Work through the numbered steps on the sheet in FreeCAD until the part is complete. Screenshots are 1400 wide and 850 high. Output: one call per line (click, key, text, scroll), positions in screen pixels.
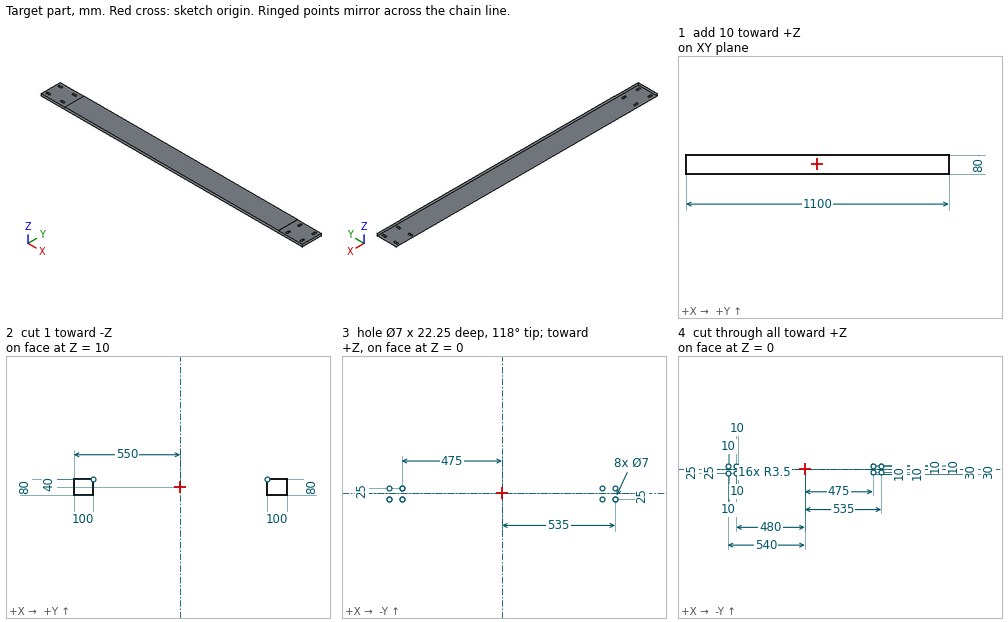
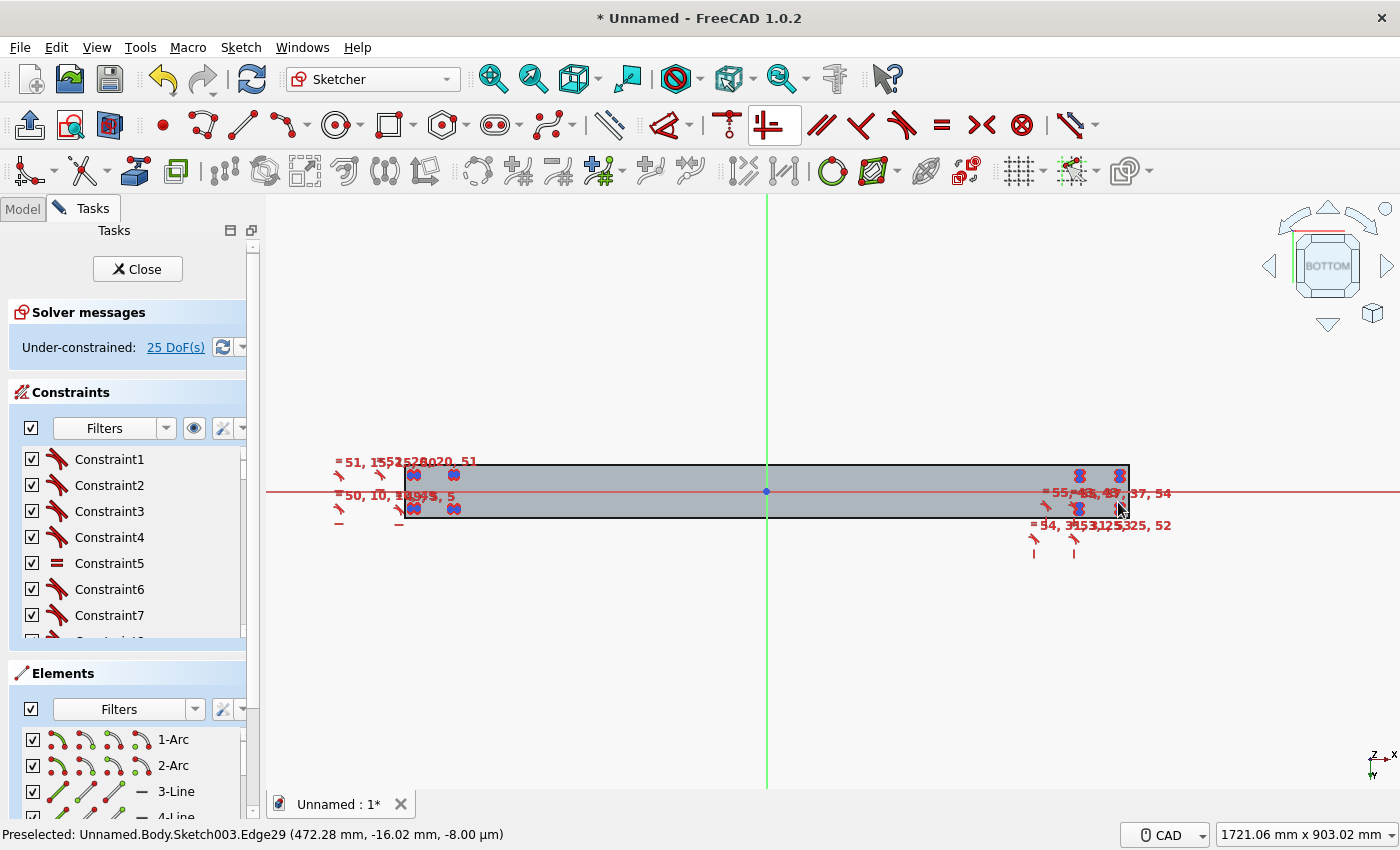
scroll(411, 508, up, 8)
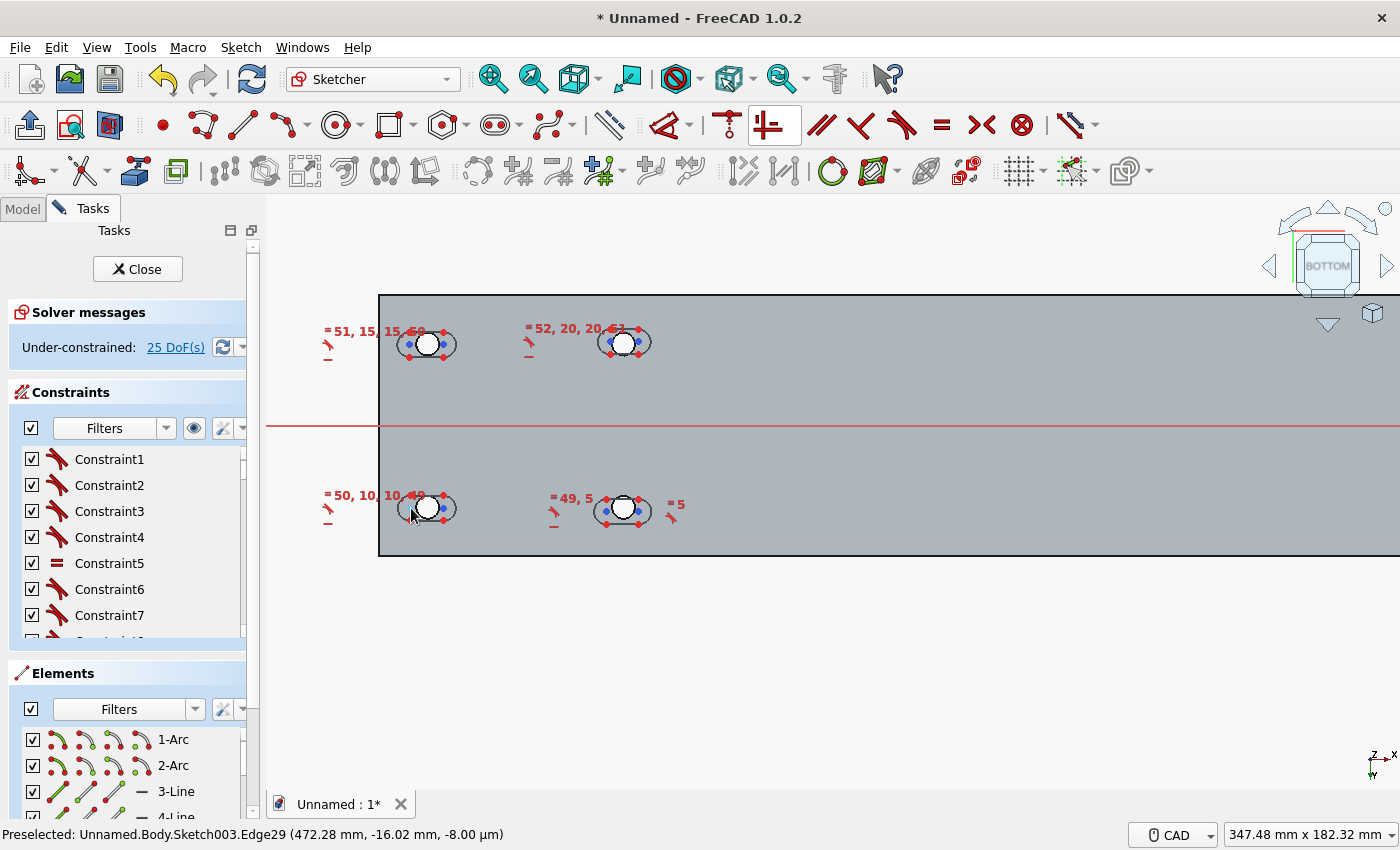
click(410, 508)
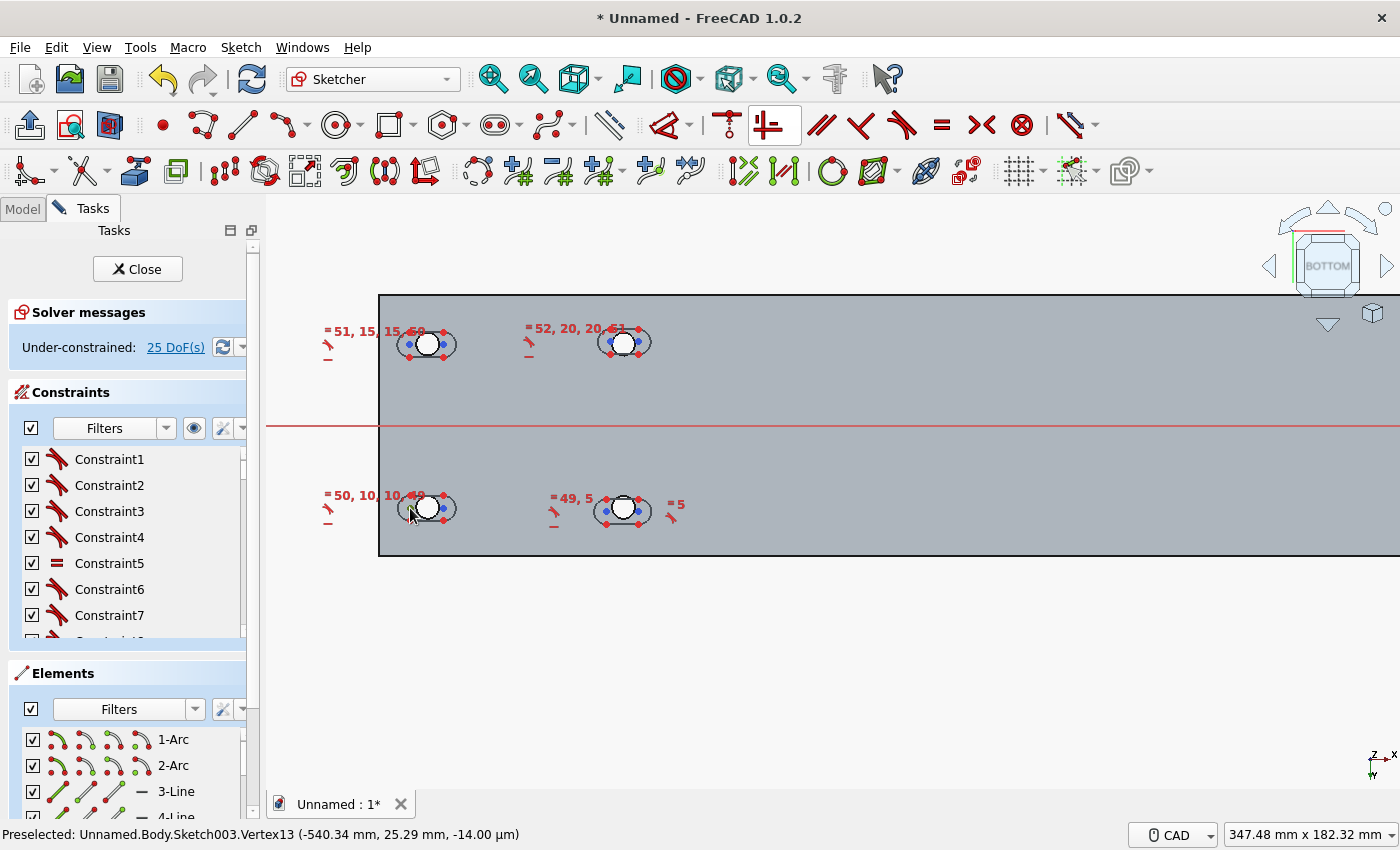
click(410, 345)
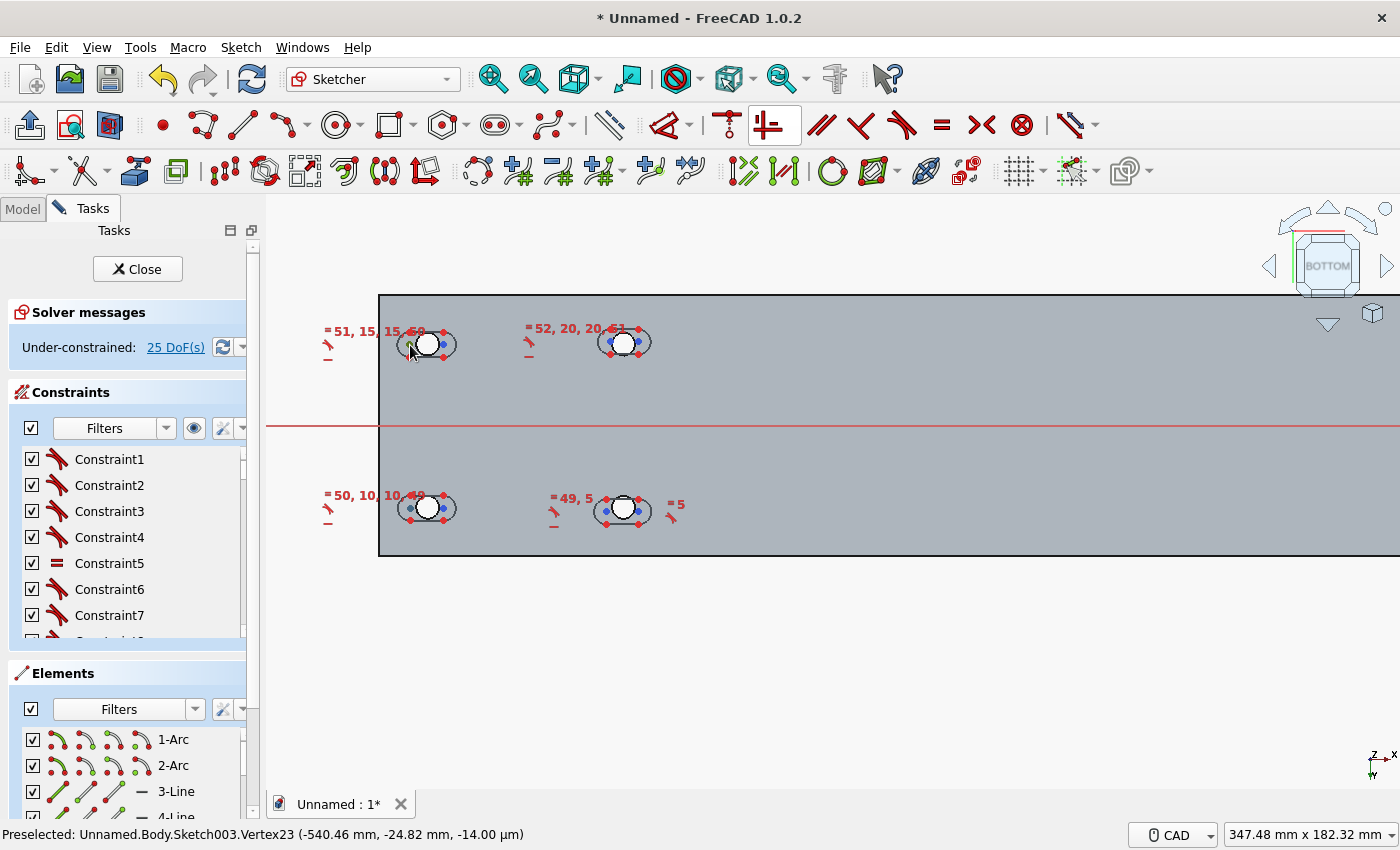
click(361, 426)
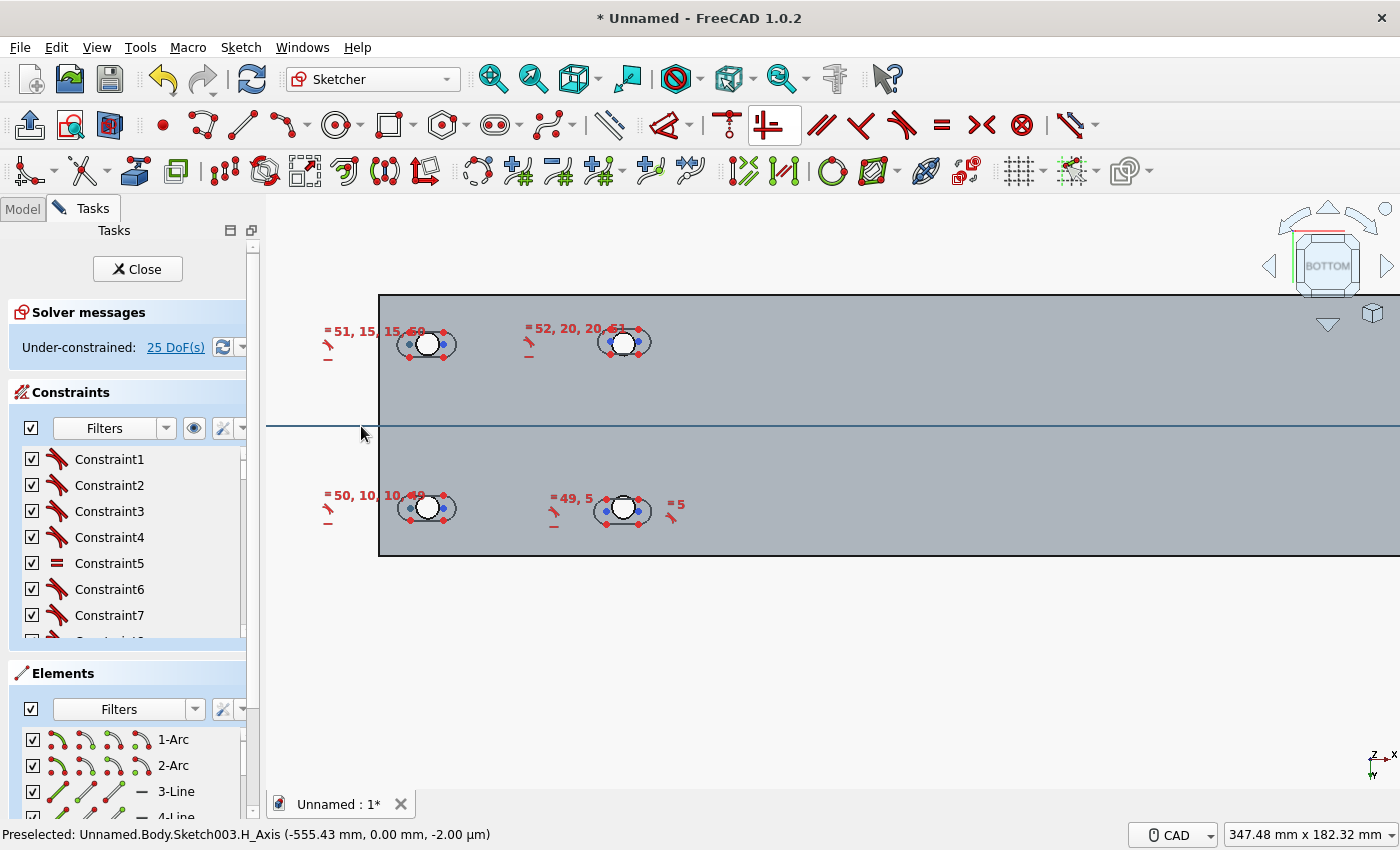
click(982, 126)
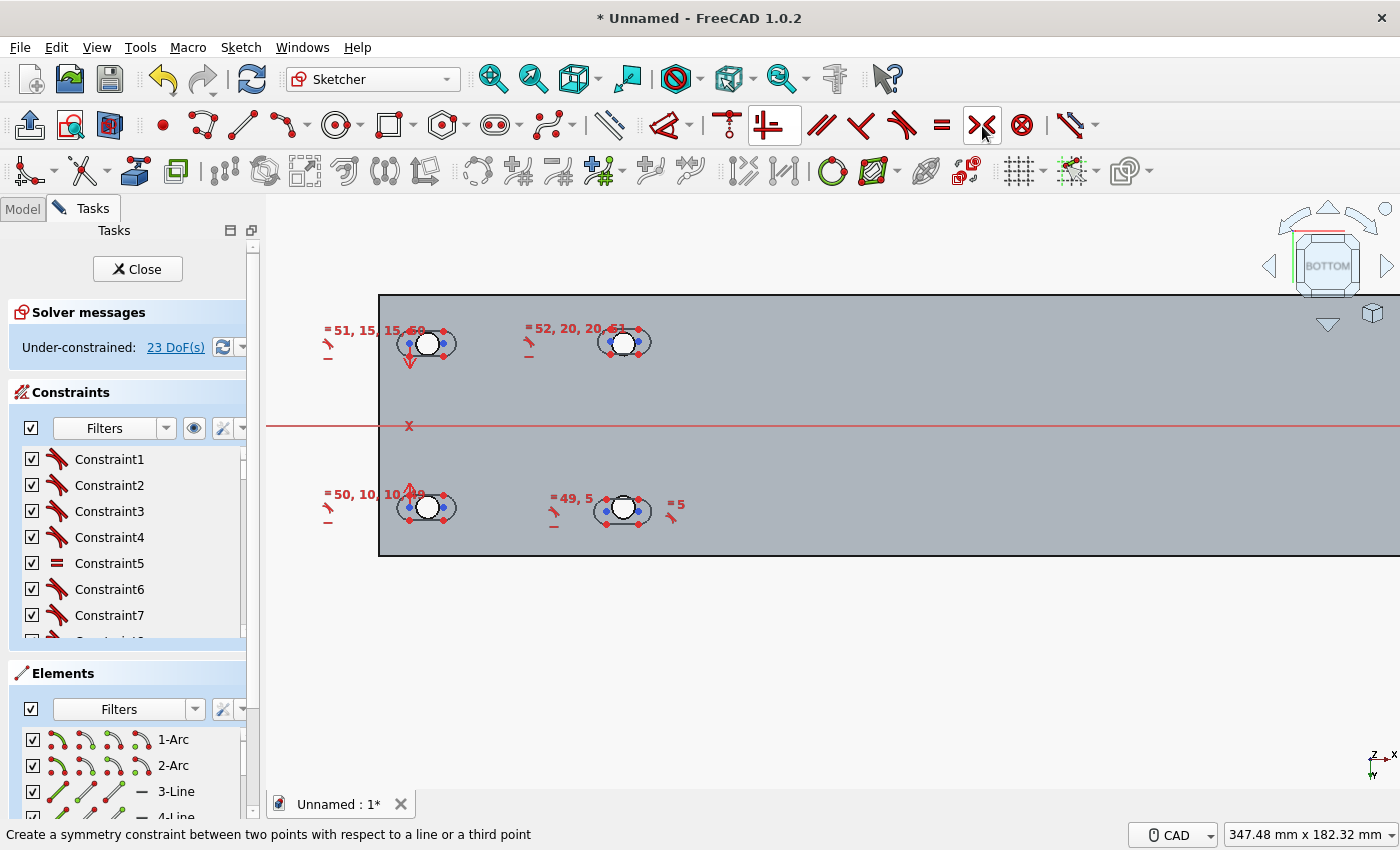
click(607, 512)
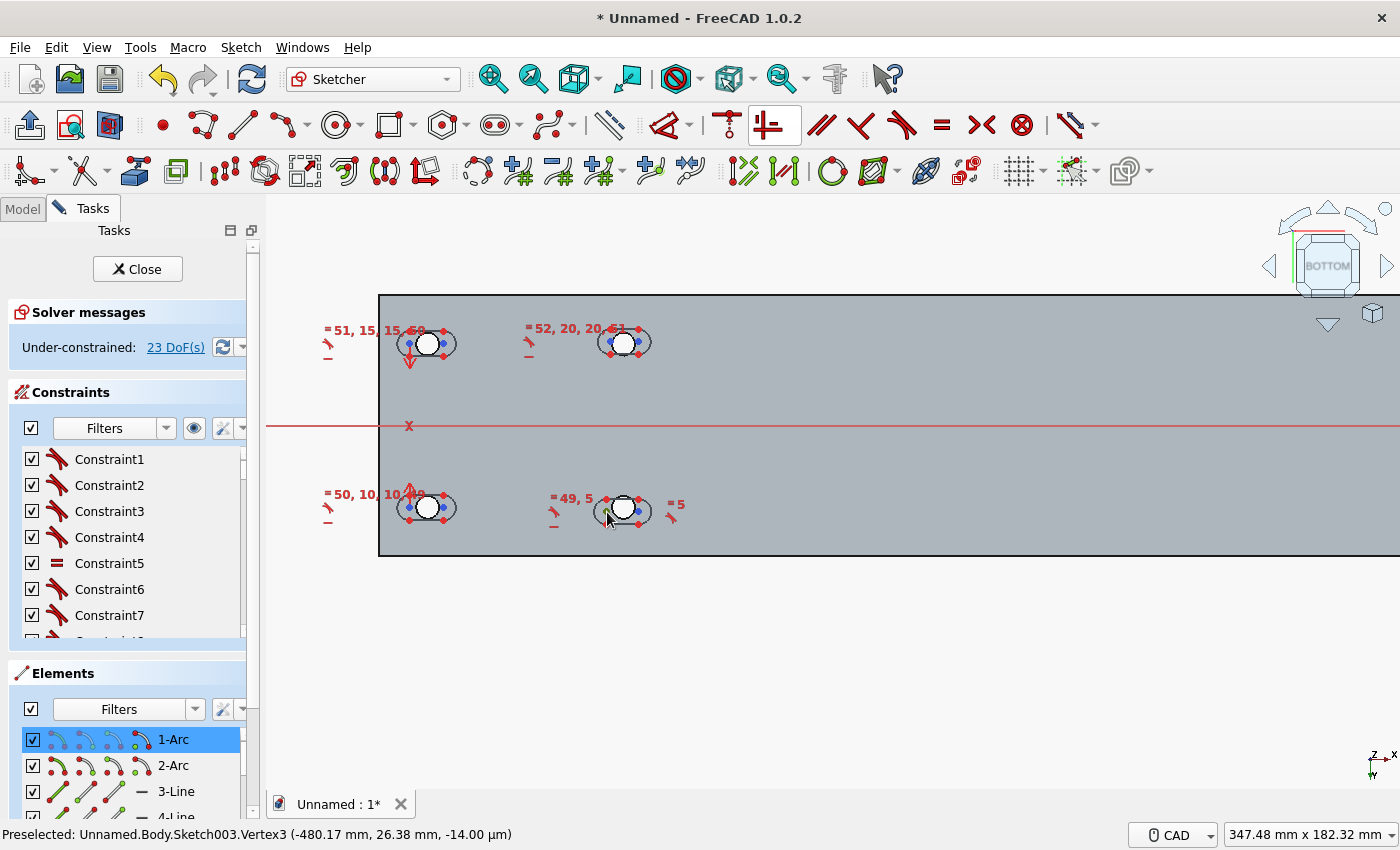
click(610, 342)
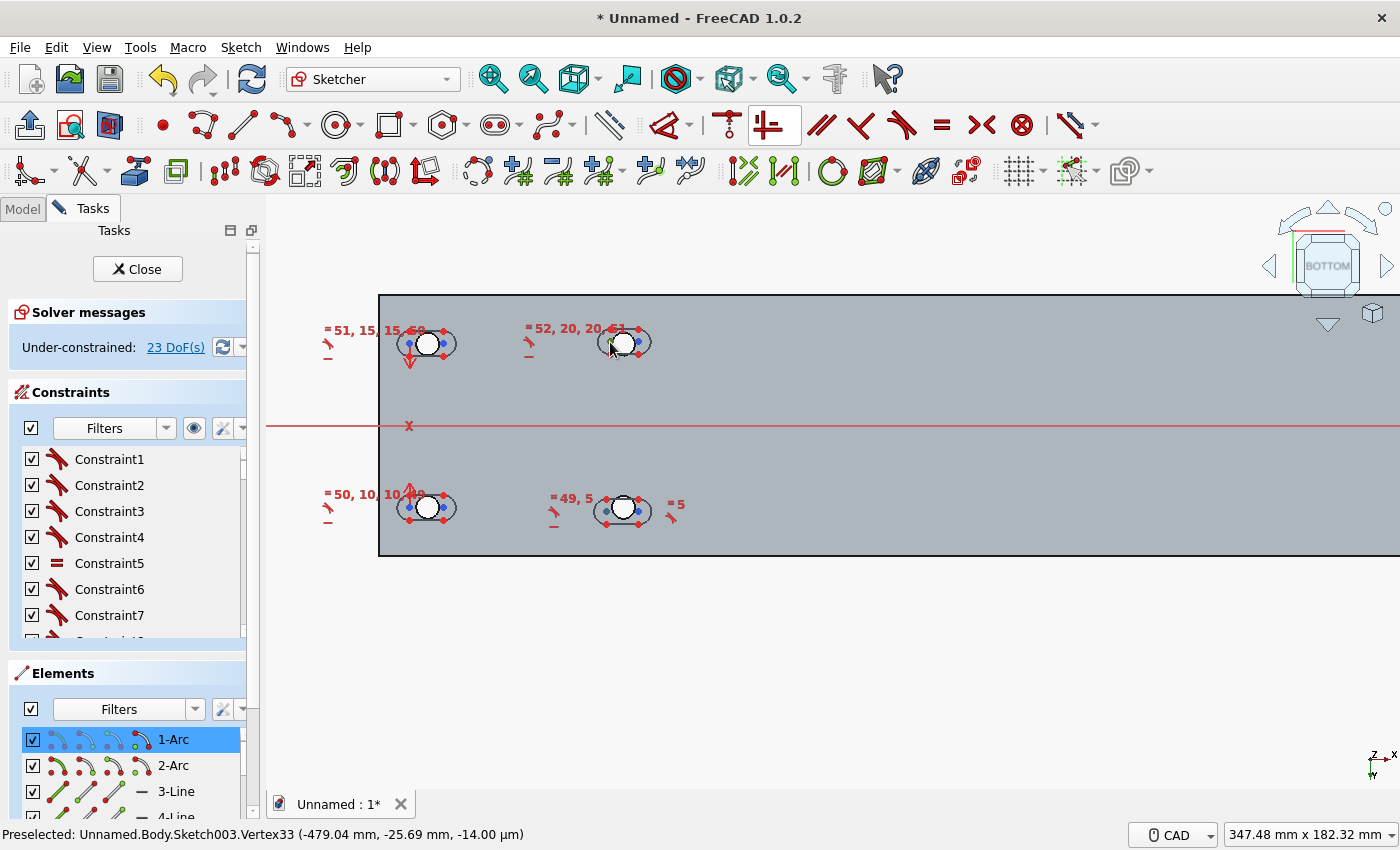
click(361, 426)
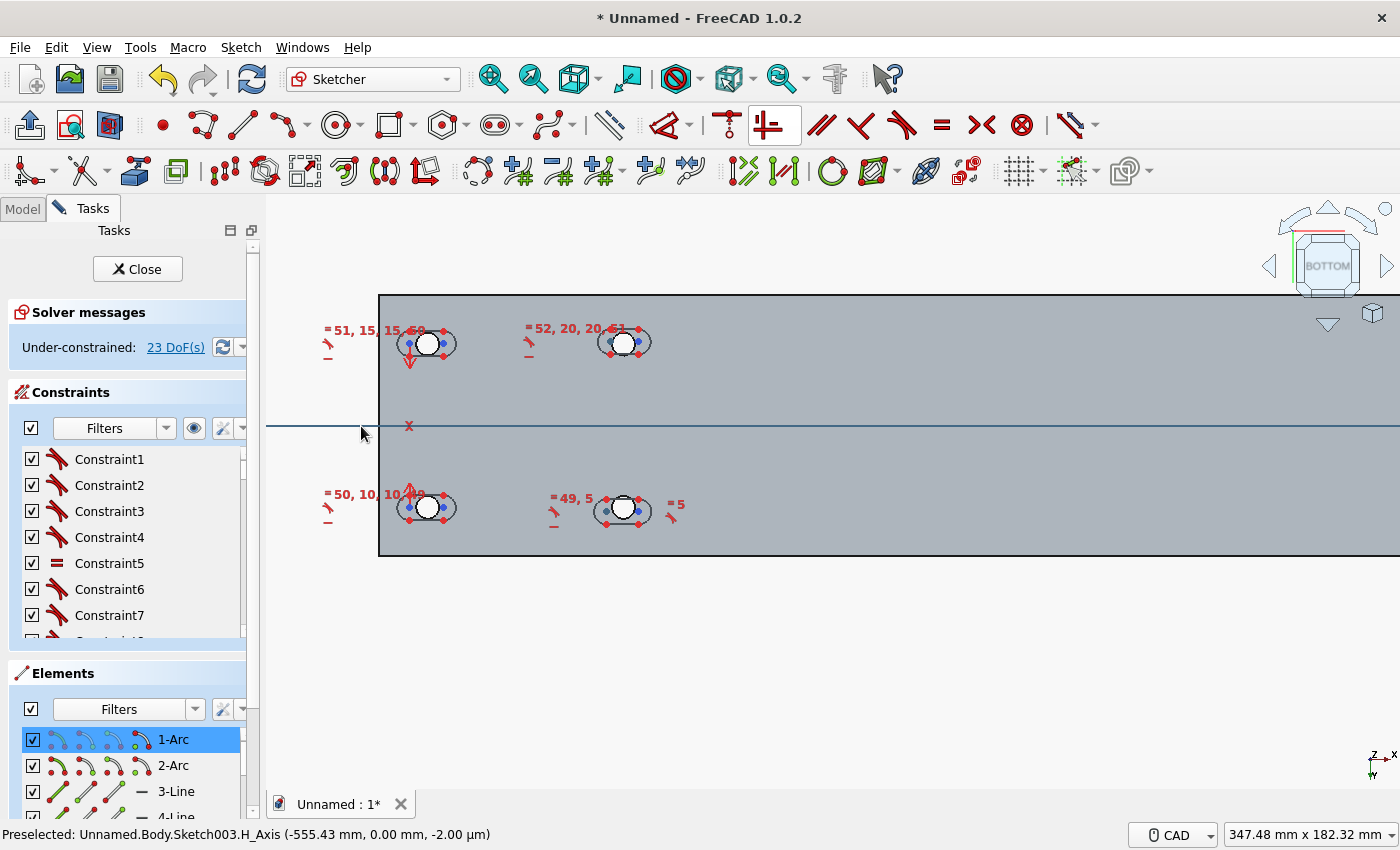
click(982, 126)